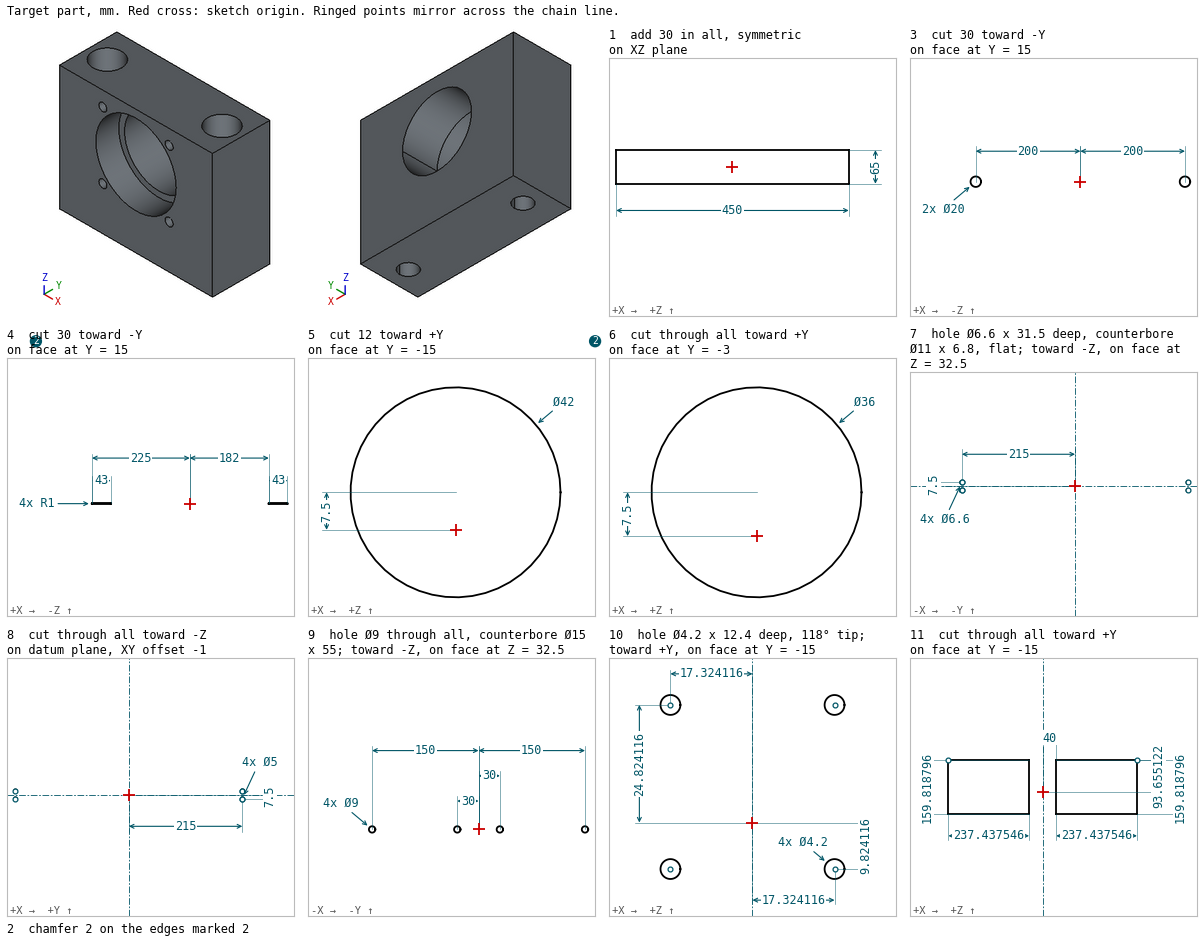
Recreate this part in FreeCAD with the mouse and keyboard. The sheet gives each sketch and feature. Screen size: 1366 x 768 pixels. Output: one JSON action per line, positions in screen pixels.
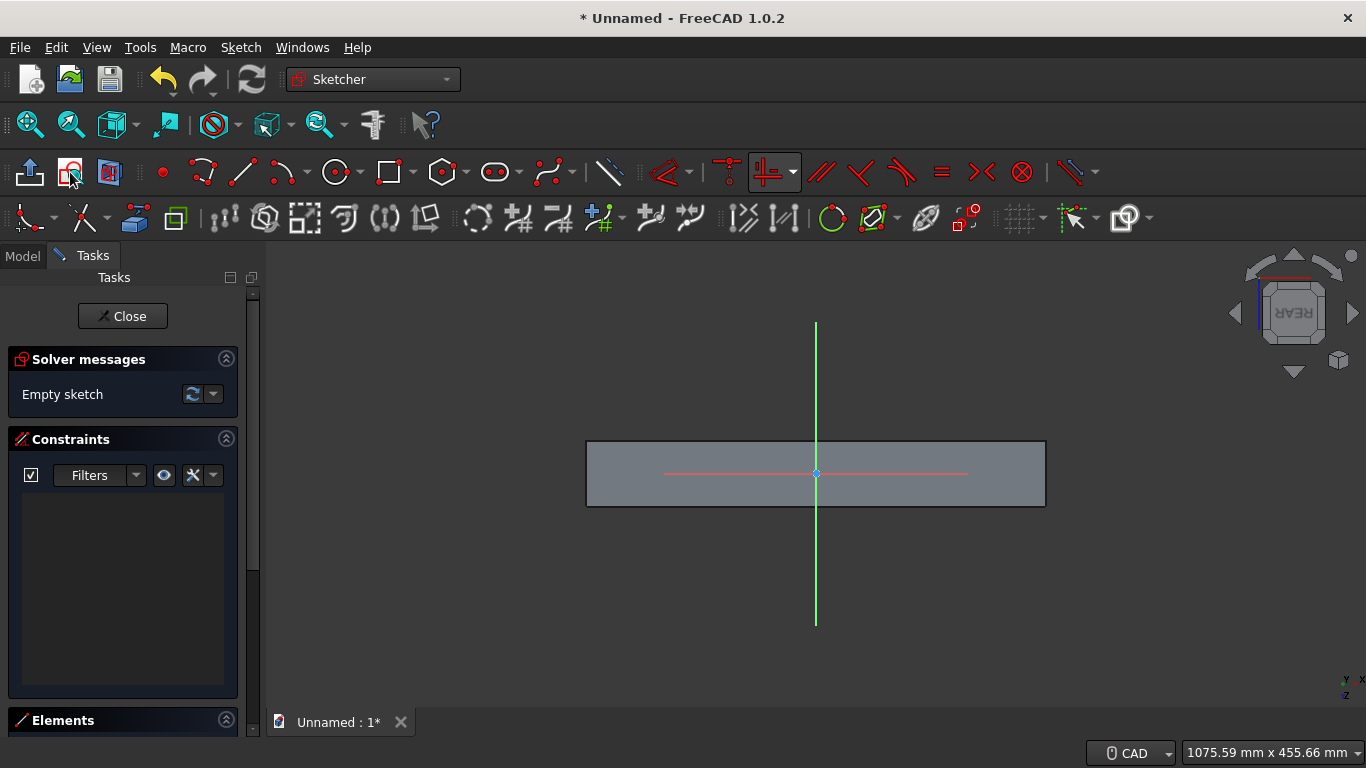
{"action": "scroll", "coordinate": [955, 474], "scroll_direction": "up", "scroll_amount": 2}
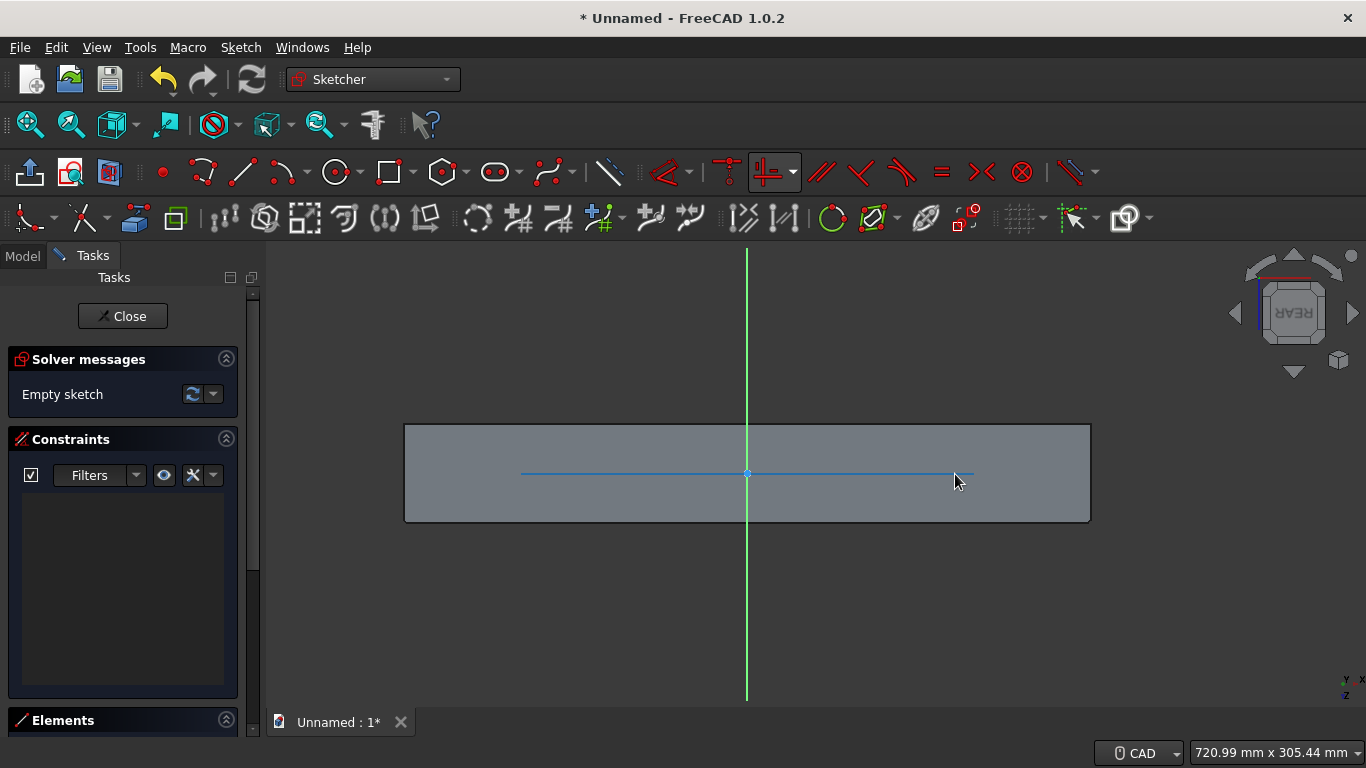
{"action": "key", "text": "g c"}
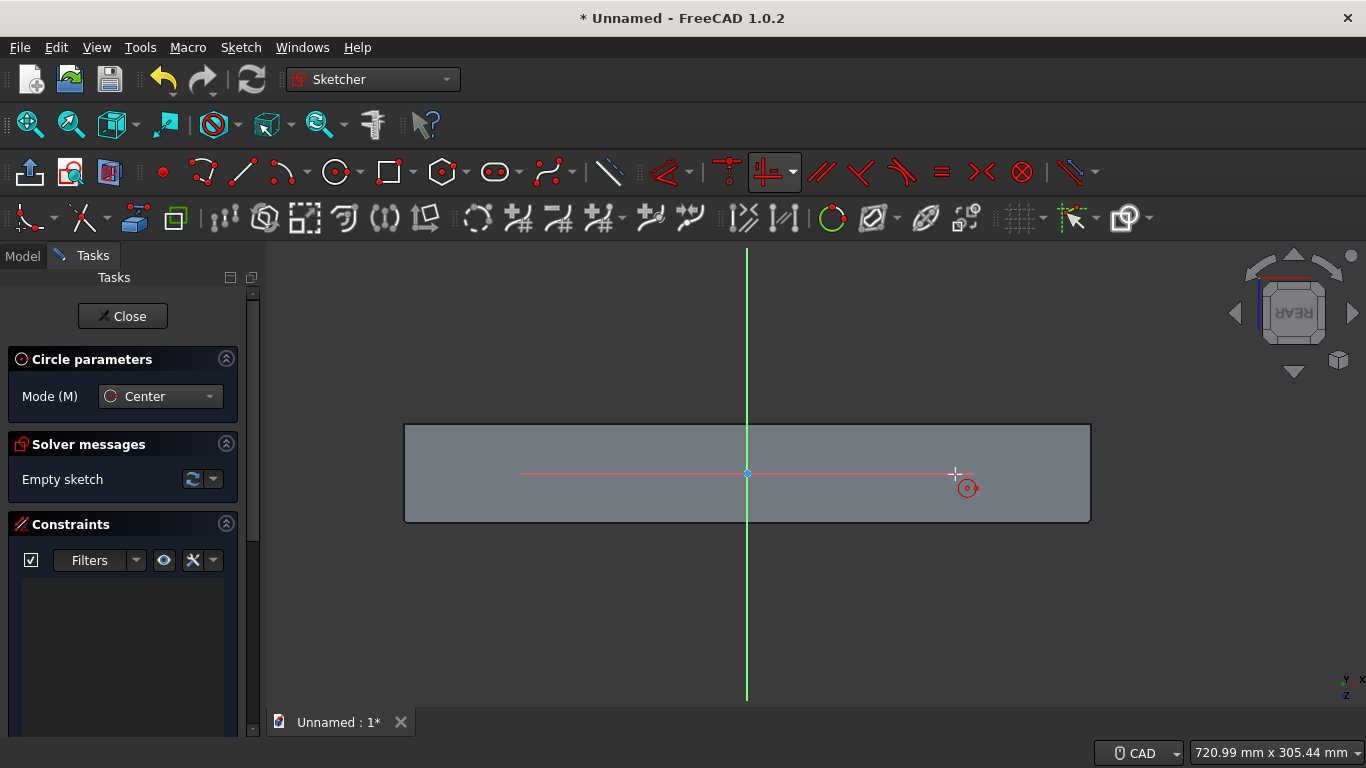
{"action": "scroll", "coordinate": [442, 474], "scroll_direction": "up", "scroll_amount": 2}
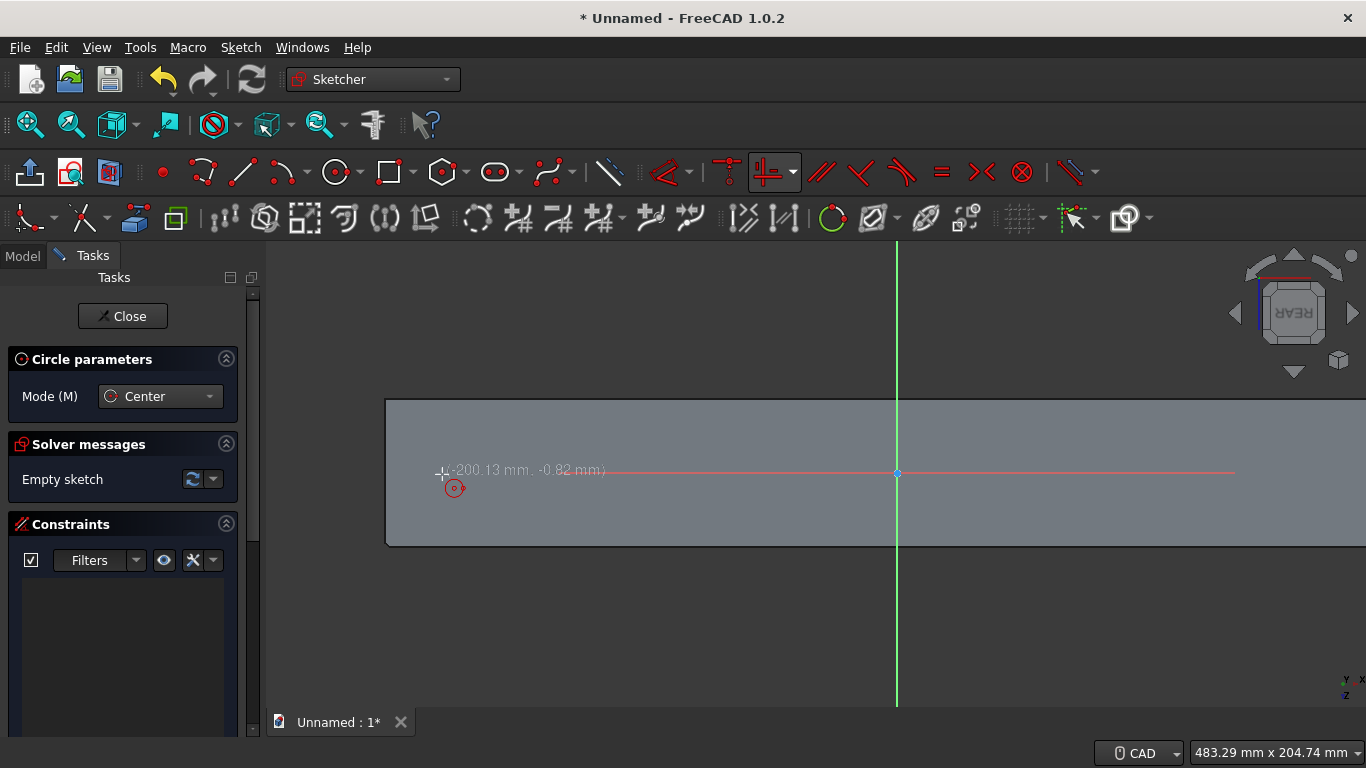
{"action": "left_click", "coordinate": [442, 473]}
{"action": "mouse_move", "coordinate": [458, 457]}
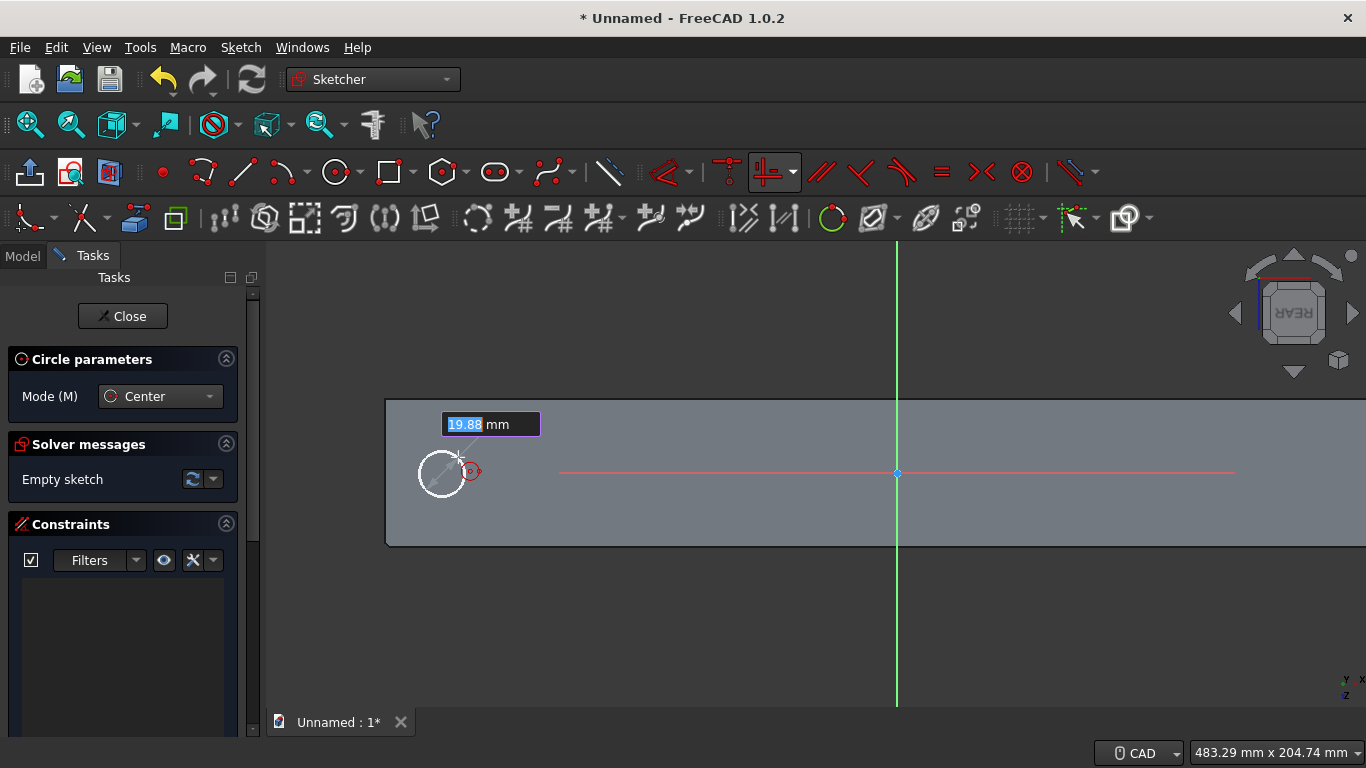
{"action": "type", "text": "20"}
{"action": "key", "text": "Return"}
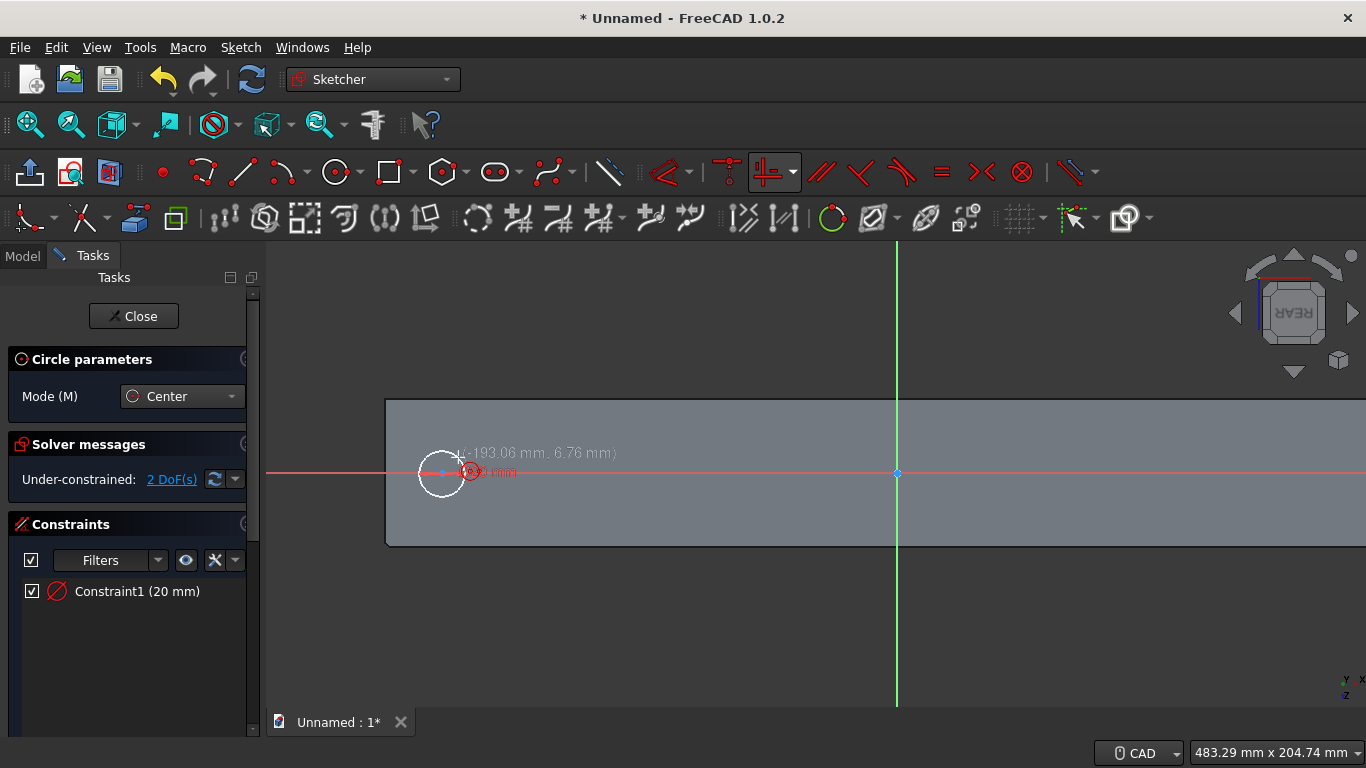
{"action": "scroll", "coordinate": [443, 475], "scroll_direction": "down", "scroll_amount": 2}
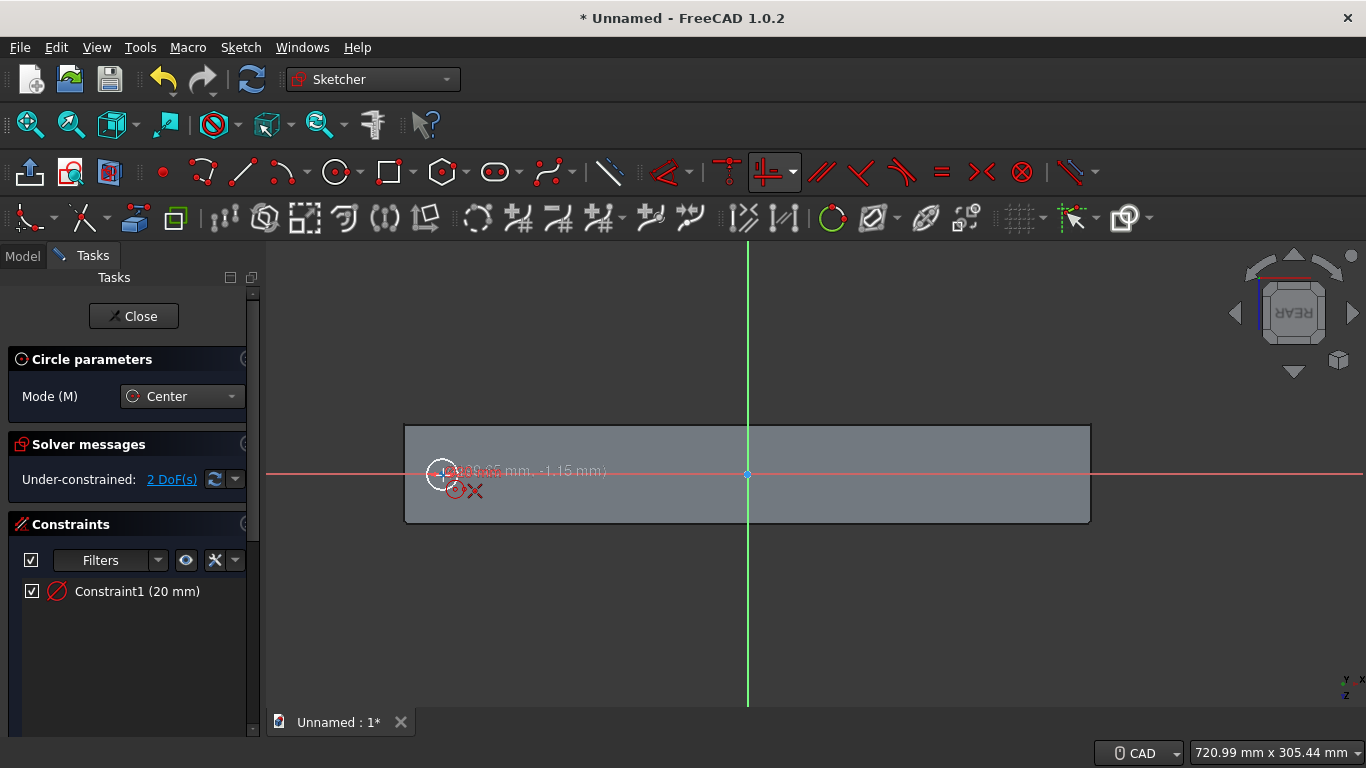
{"action": "scroll", "coordinate": [1053, 474], "scroll_direction": "up", "scroll_amount": 2}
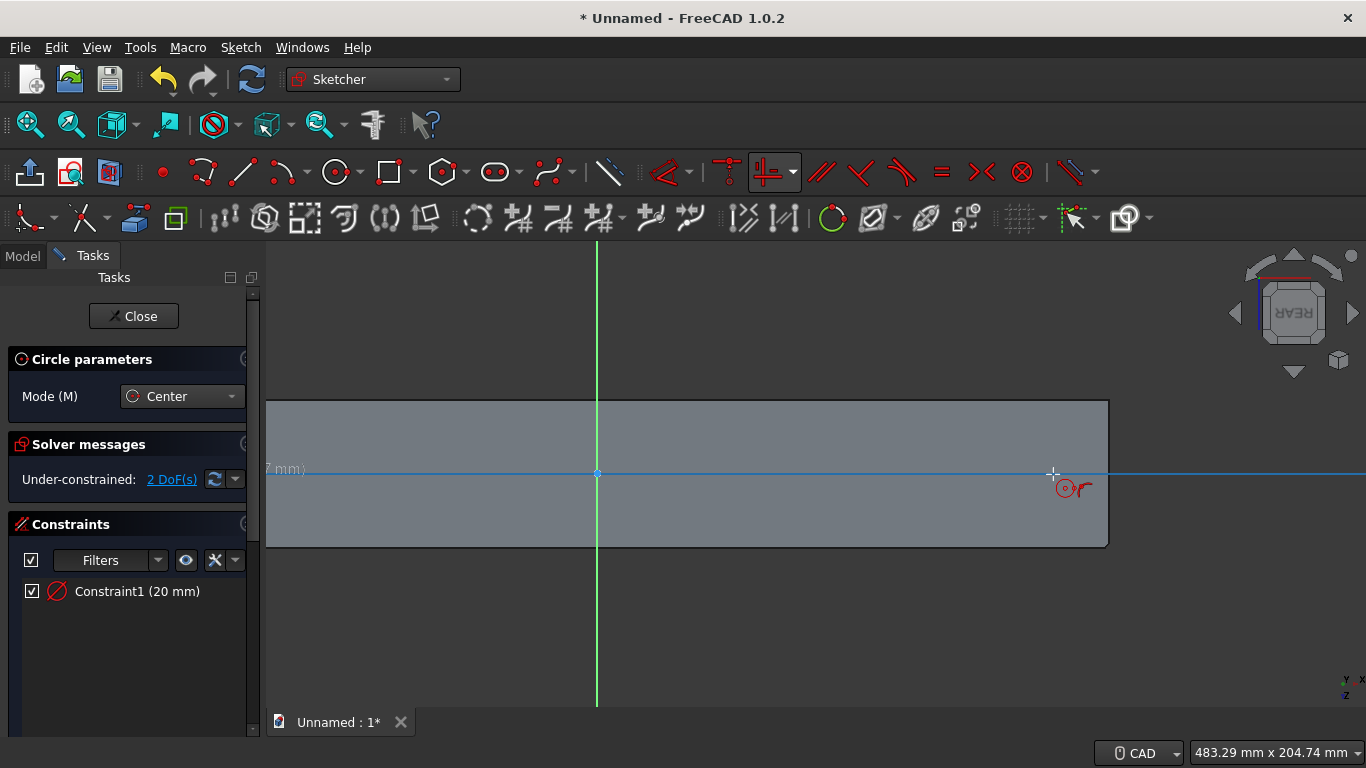
{"action": "left_click", "coordinate": [1052, 474]}
{"action": "mouse_move", "coordinate": [1068, 458]}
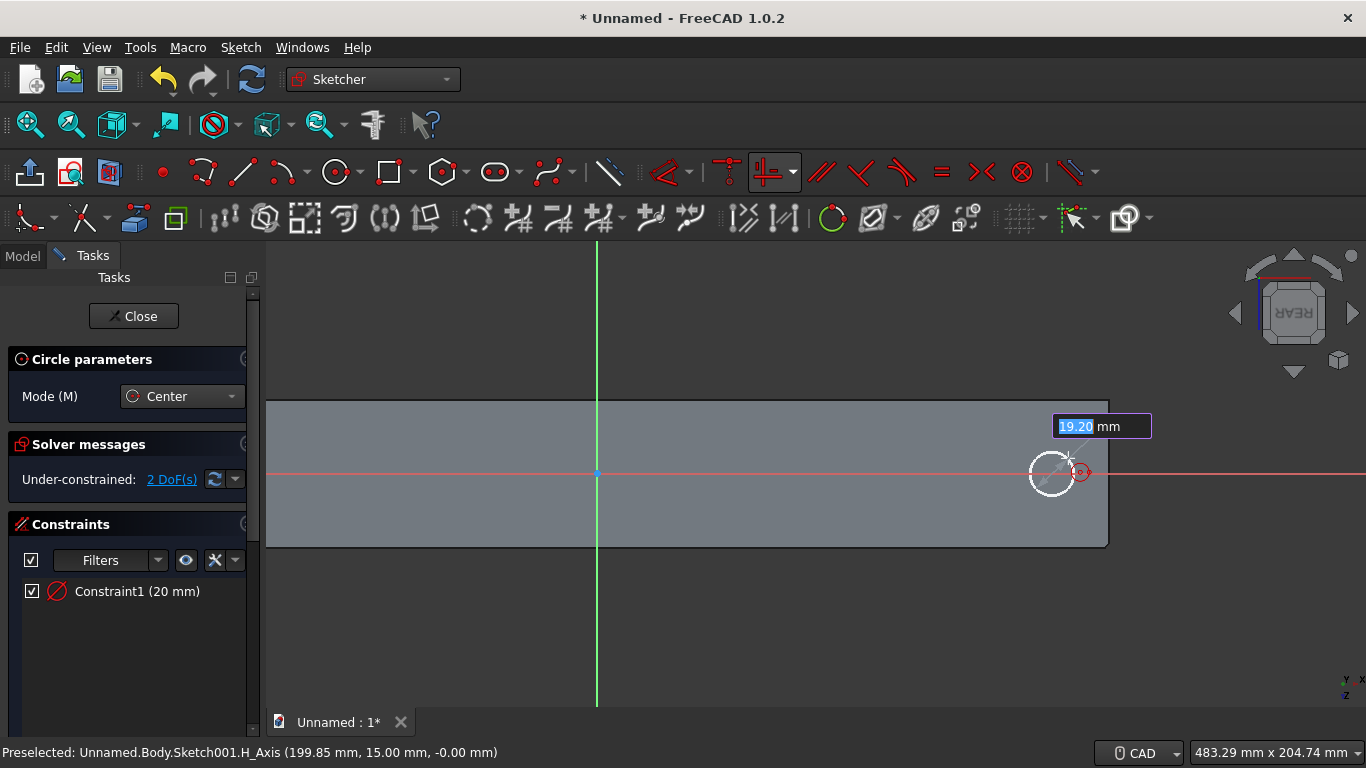
{"action": "type", "text": "20"}
{"action": "key", "text": "Return"}
{"action": "key", "text": "Escape"}